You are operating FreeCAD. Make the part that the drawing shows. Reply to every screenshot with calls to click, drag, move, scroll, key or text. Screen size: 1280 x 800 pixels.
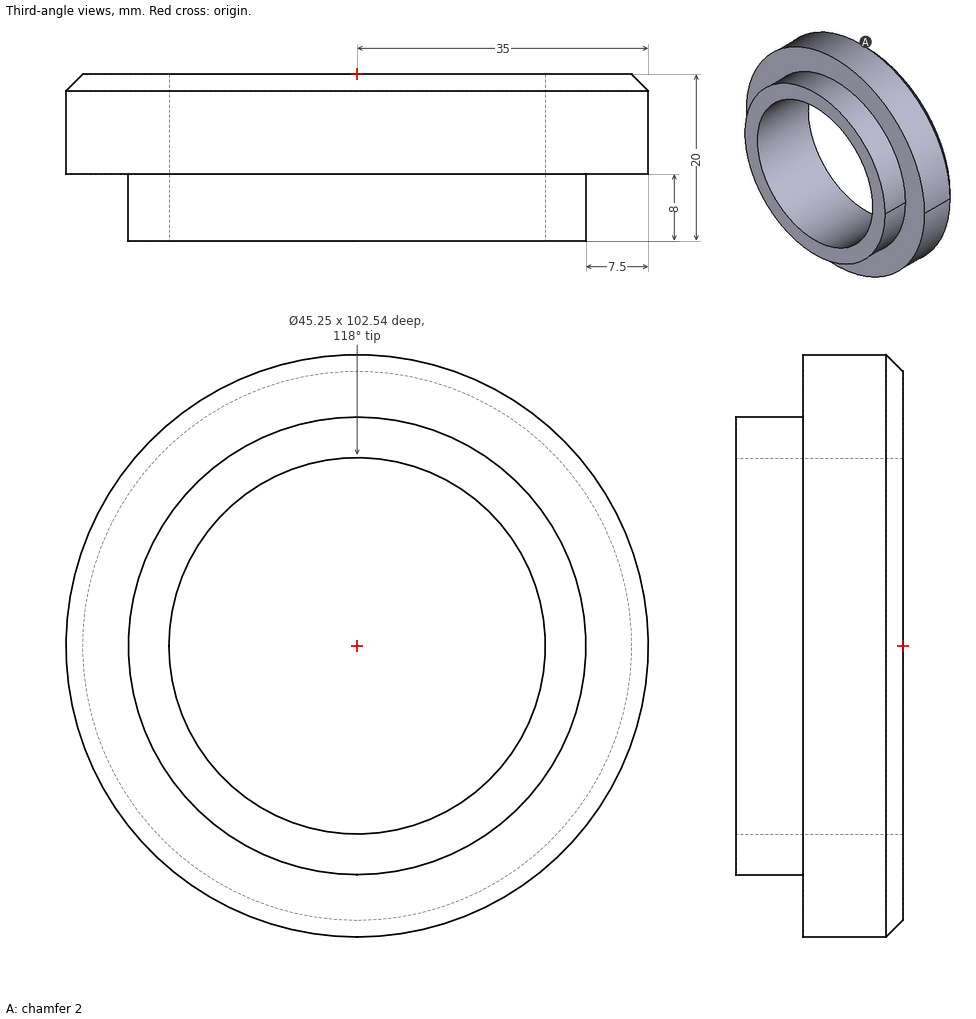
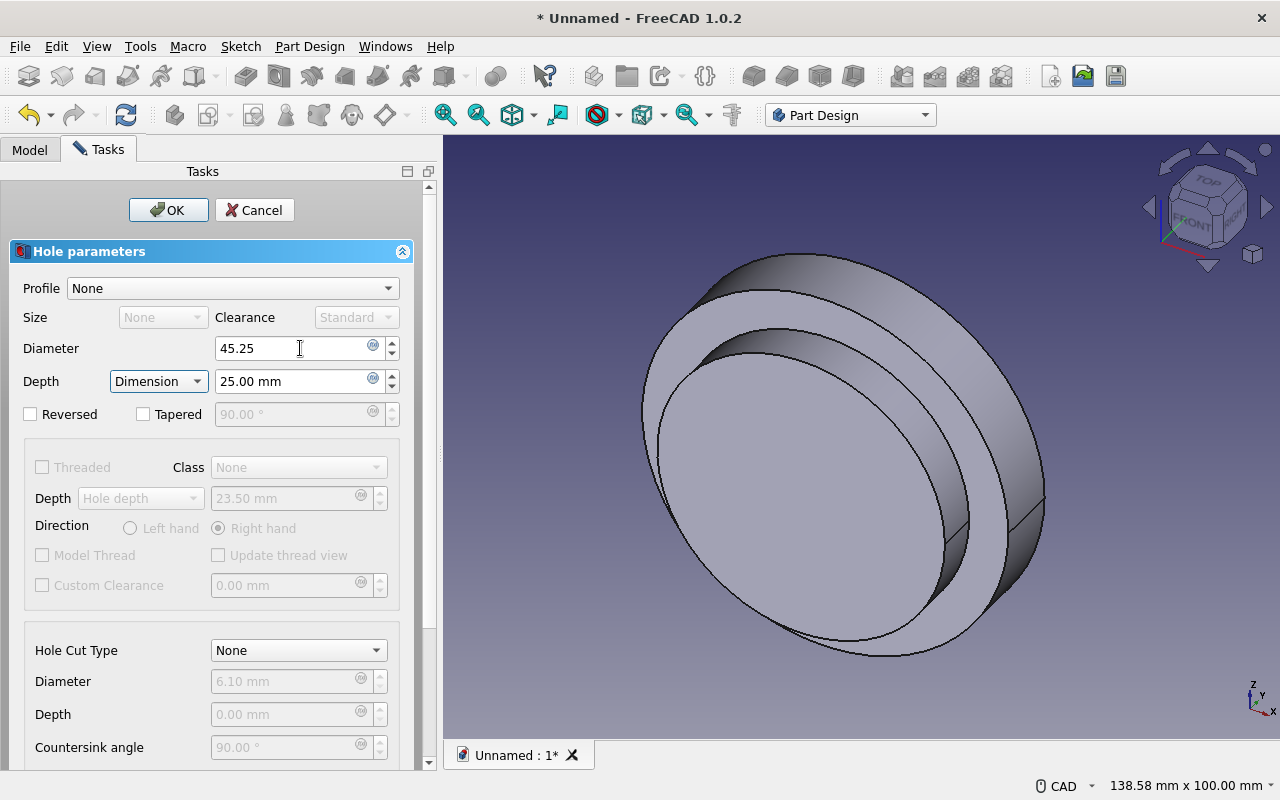
triple_click(300, 382)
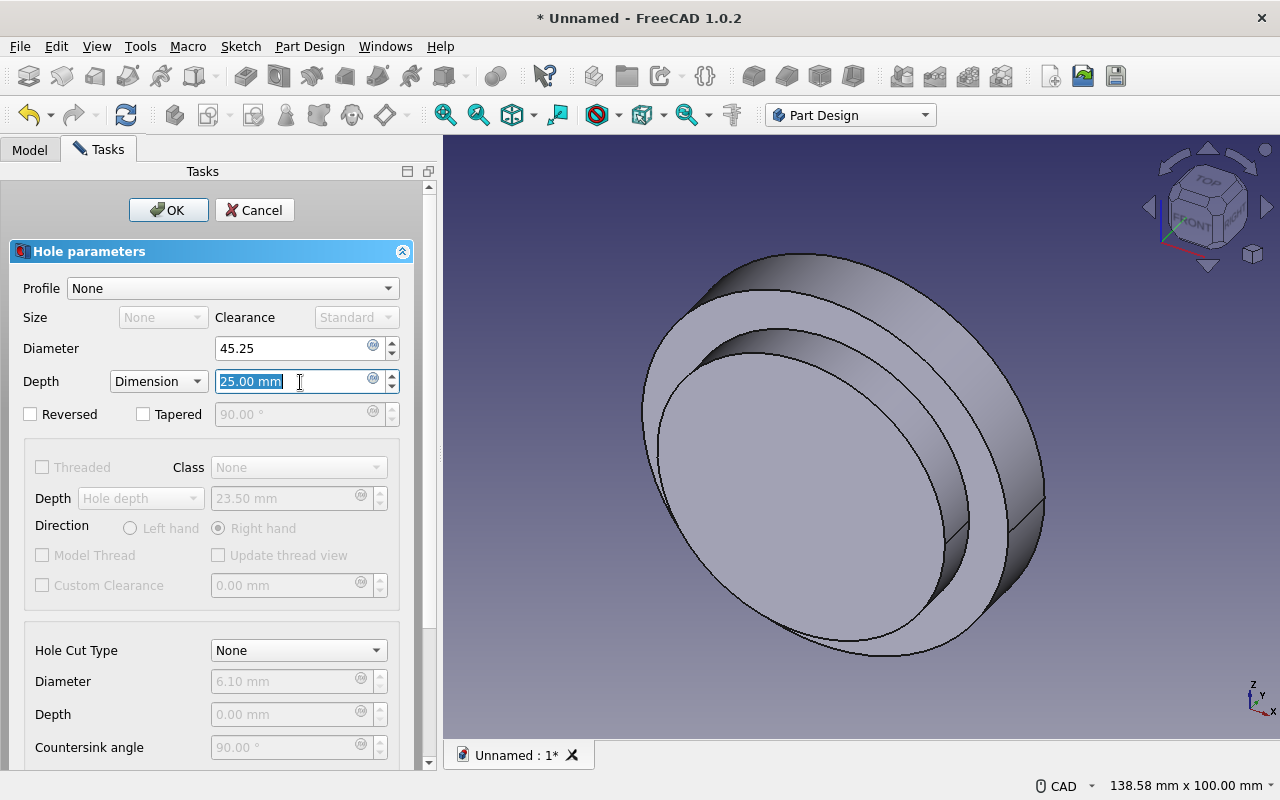
text(102.54)
key(Tab)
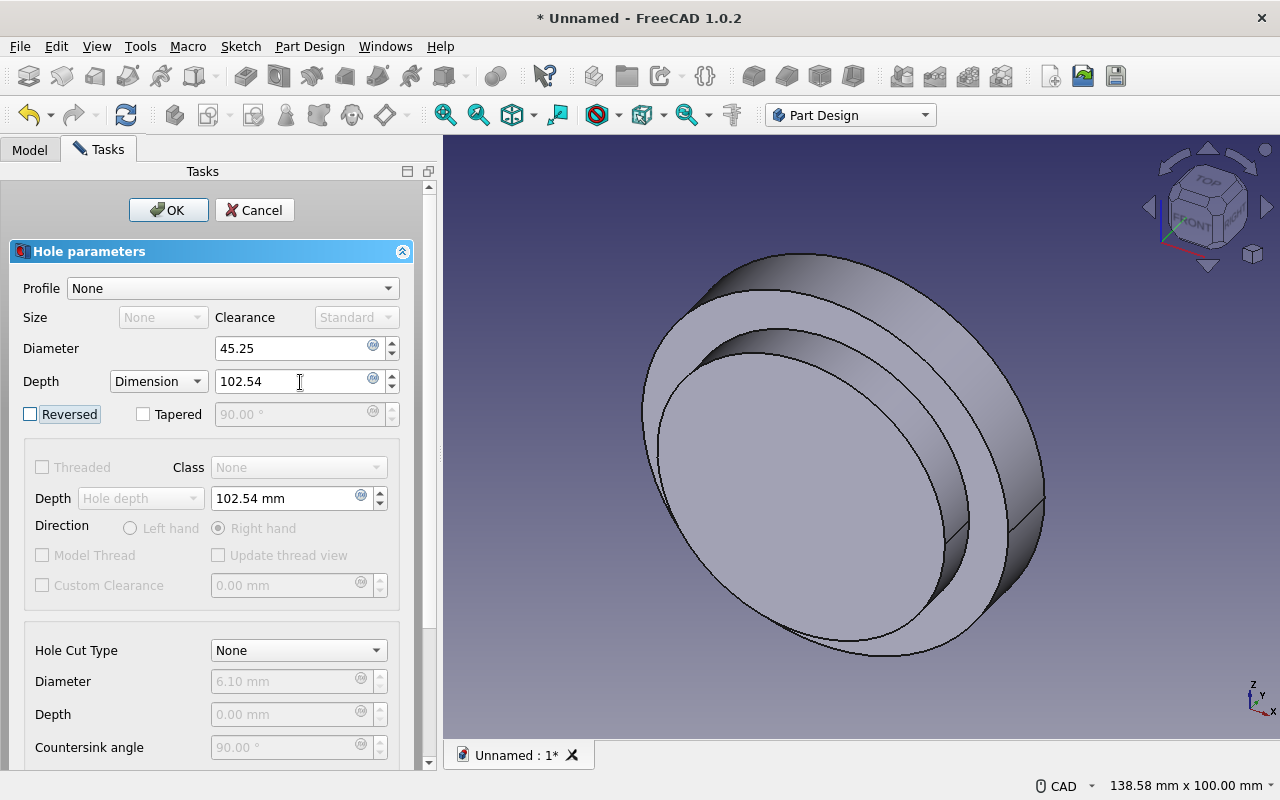
click(31, 414)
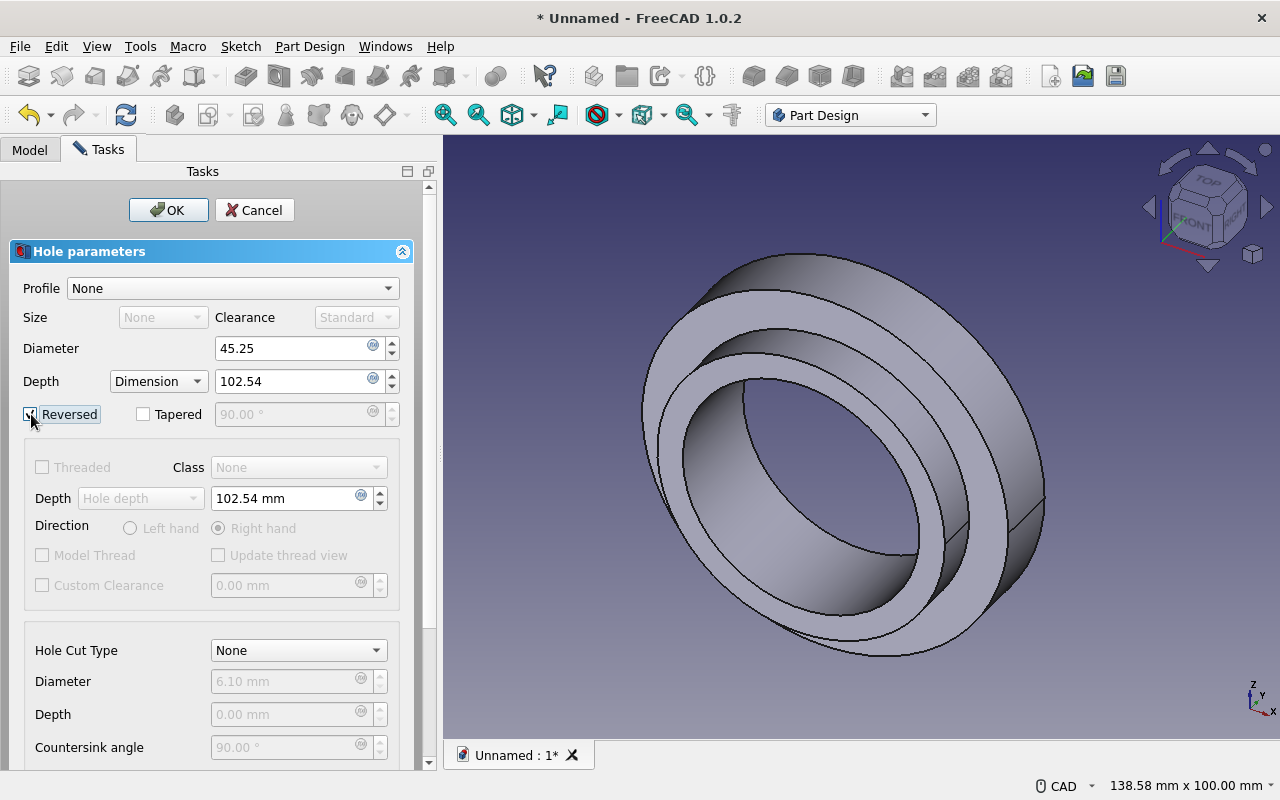
click(169, 210)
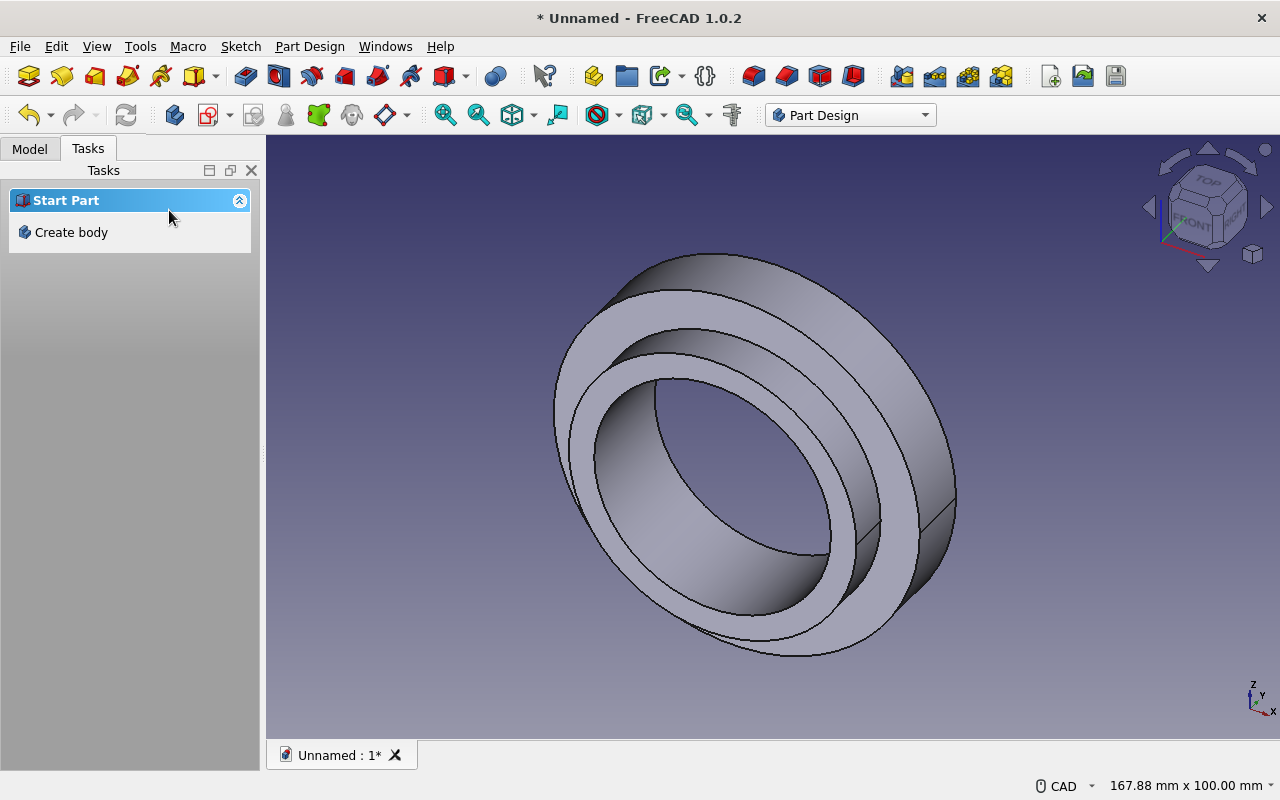
key(0)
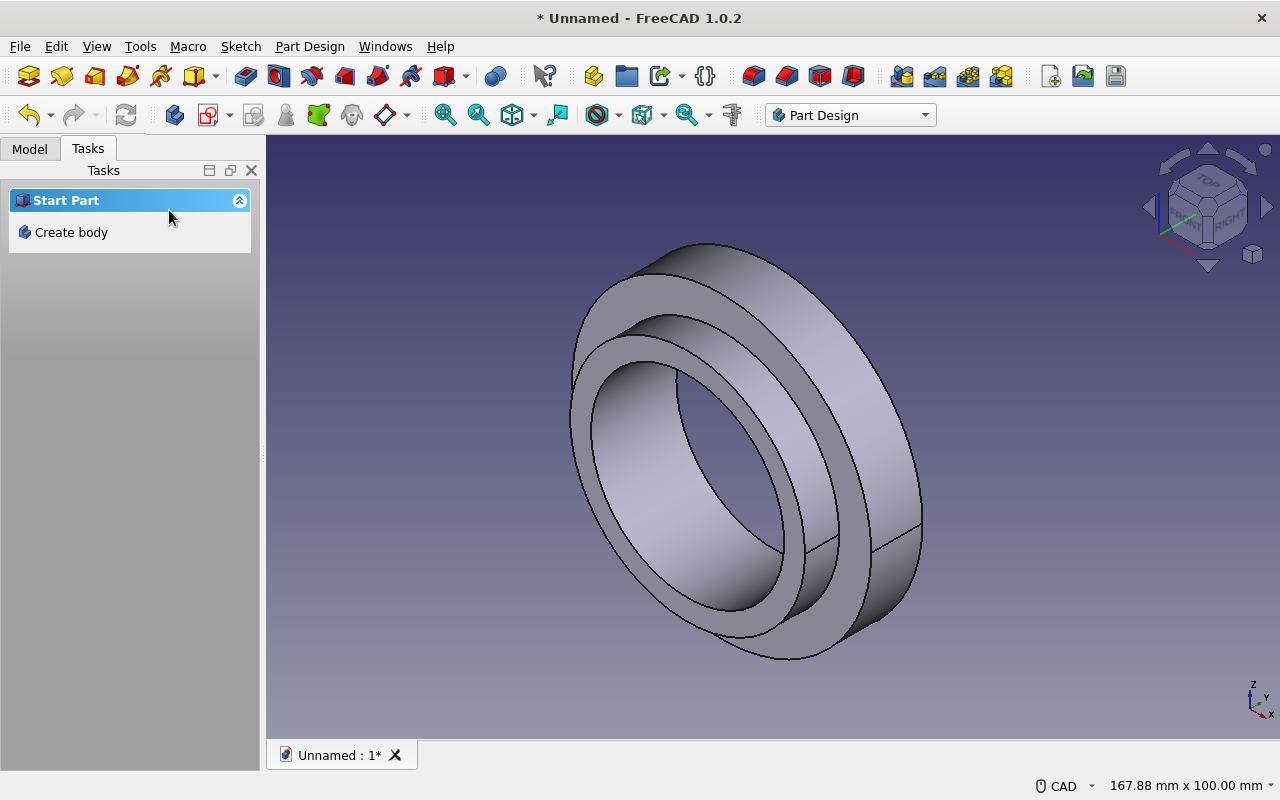
click(446, 116)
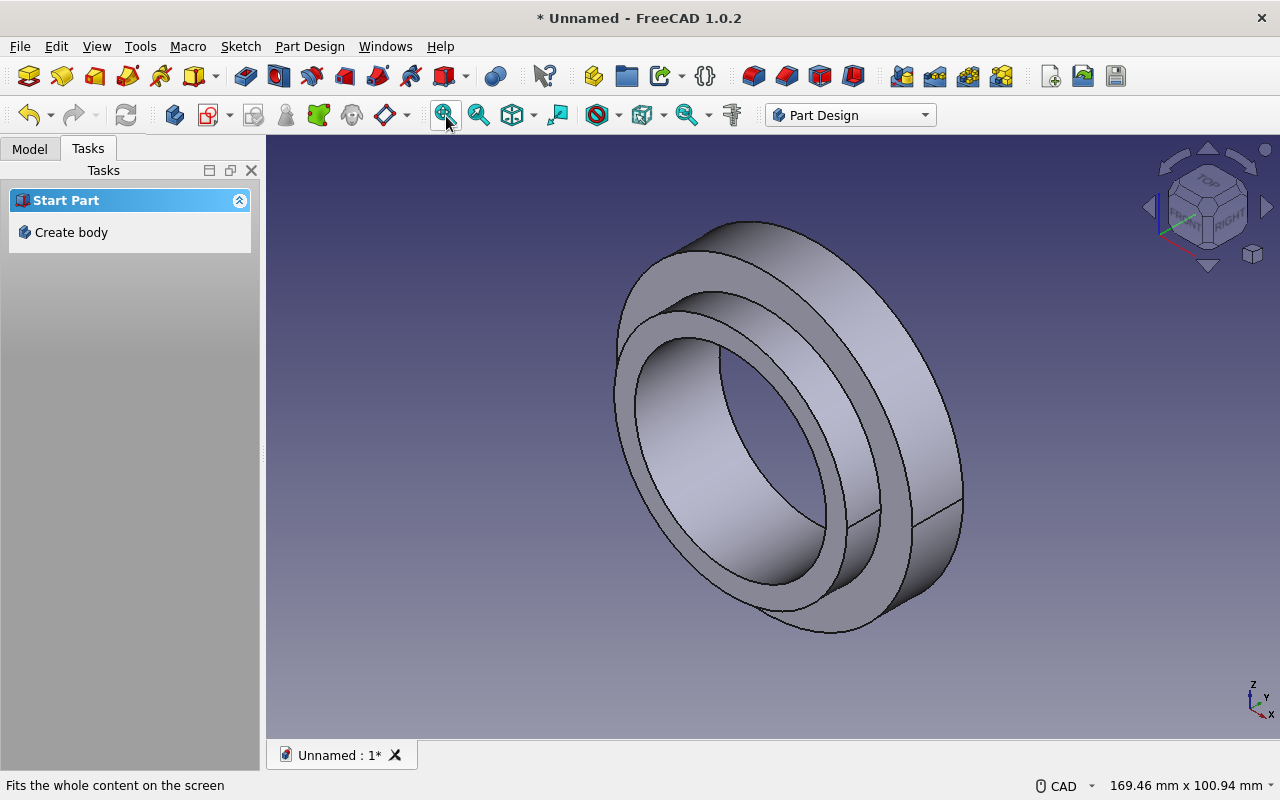
click(769, 222)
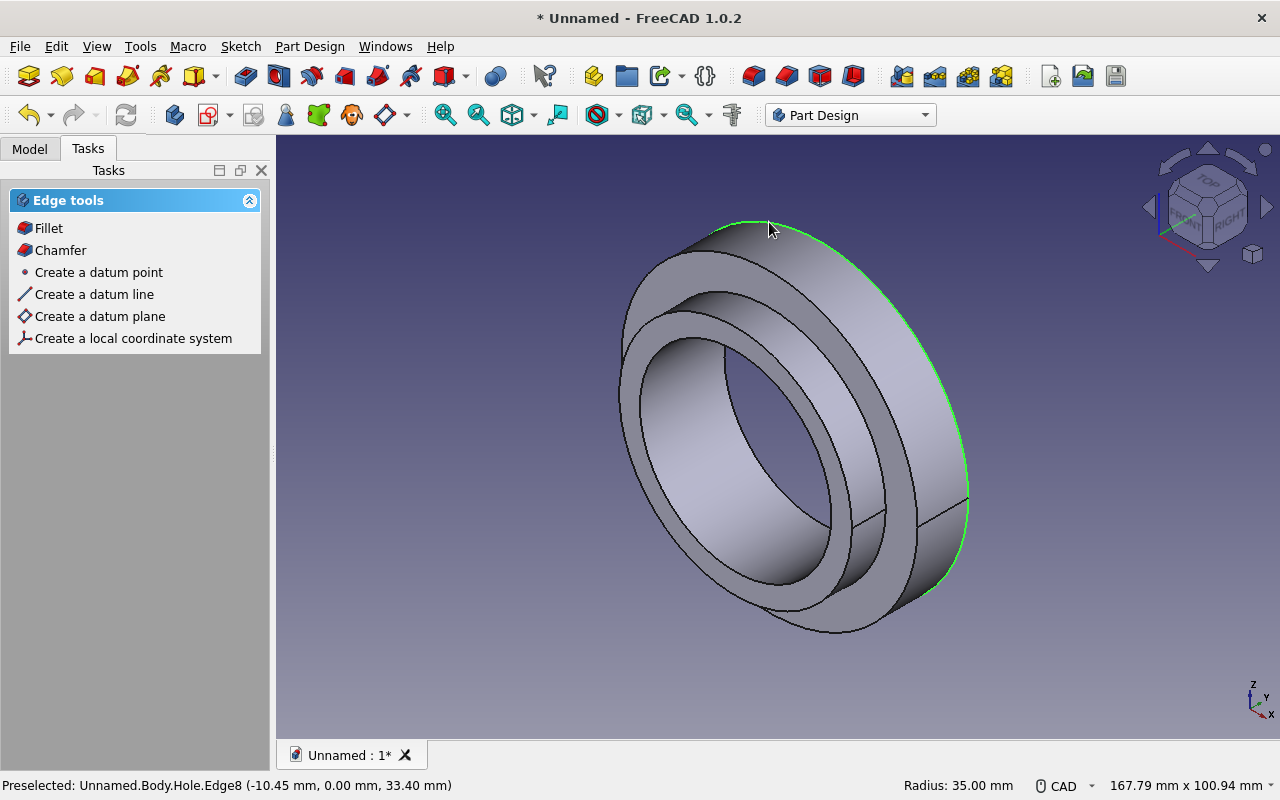
click(787, 76)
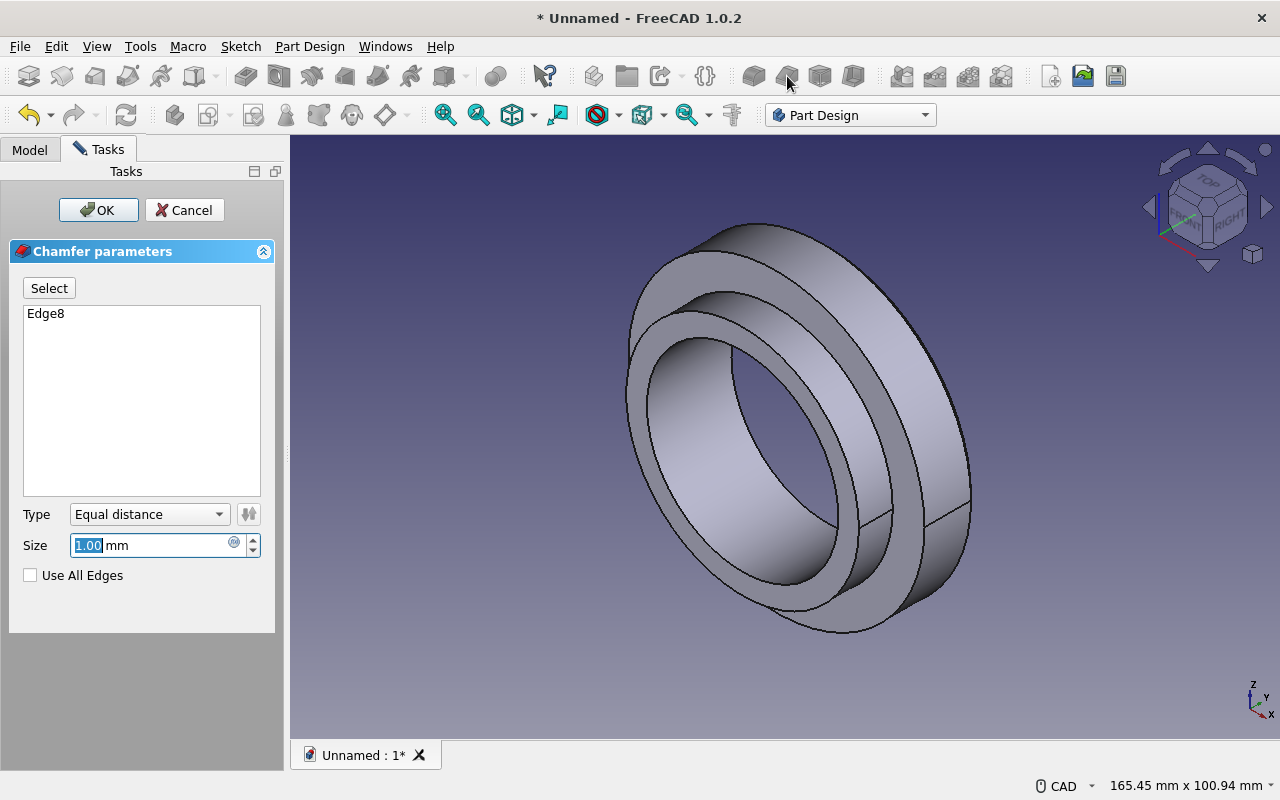
text(2)
key(Tab)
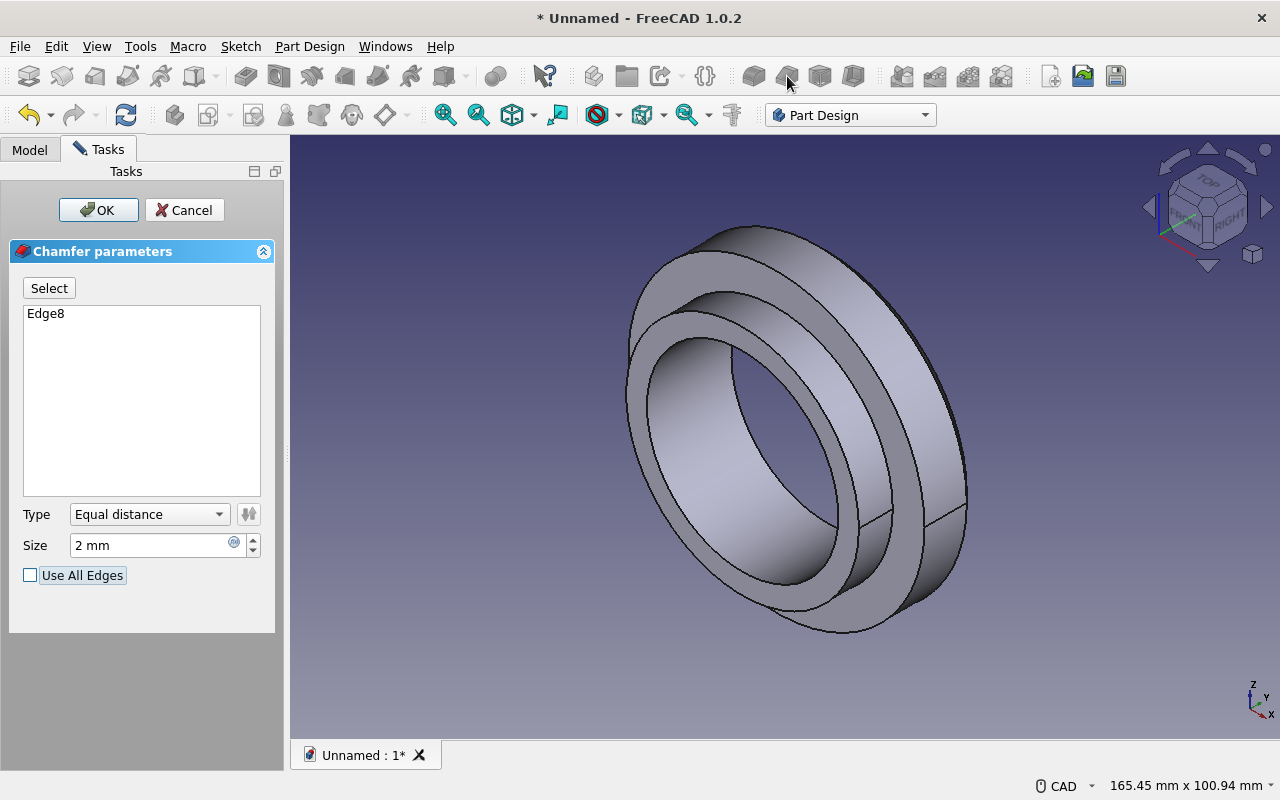
click(99, 210)